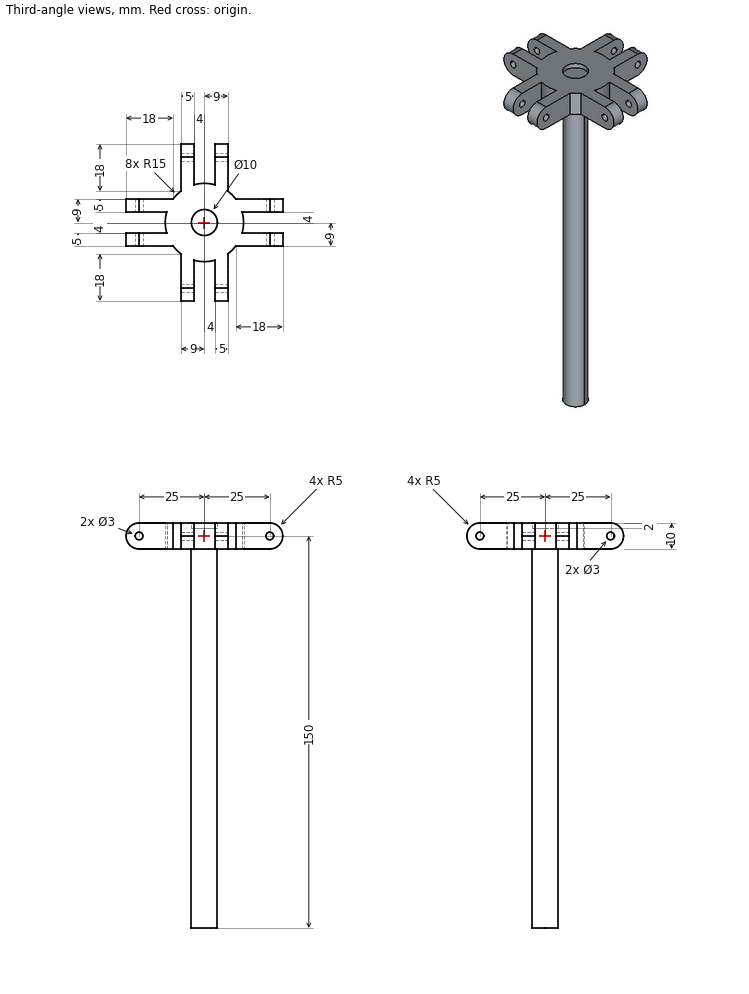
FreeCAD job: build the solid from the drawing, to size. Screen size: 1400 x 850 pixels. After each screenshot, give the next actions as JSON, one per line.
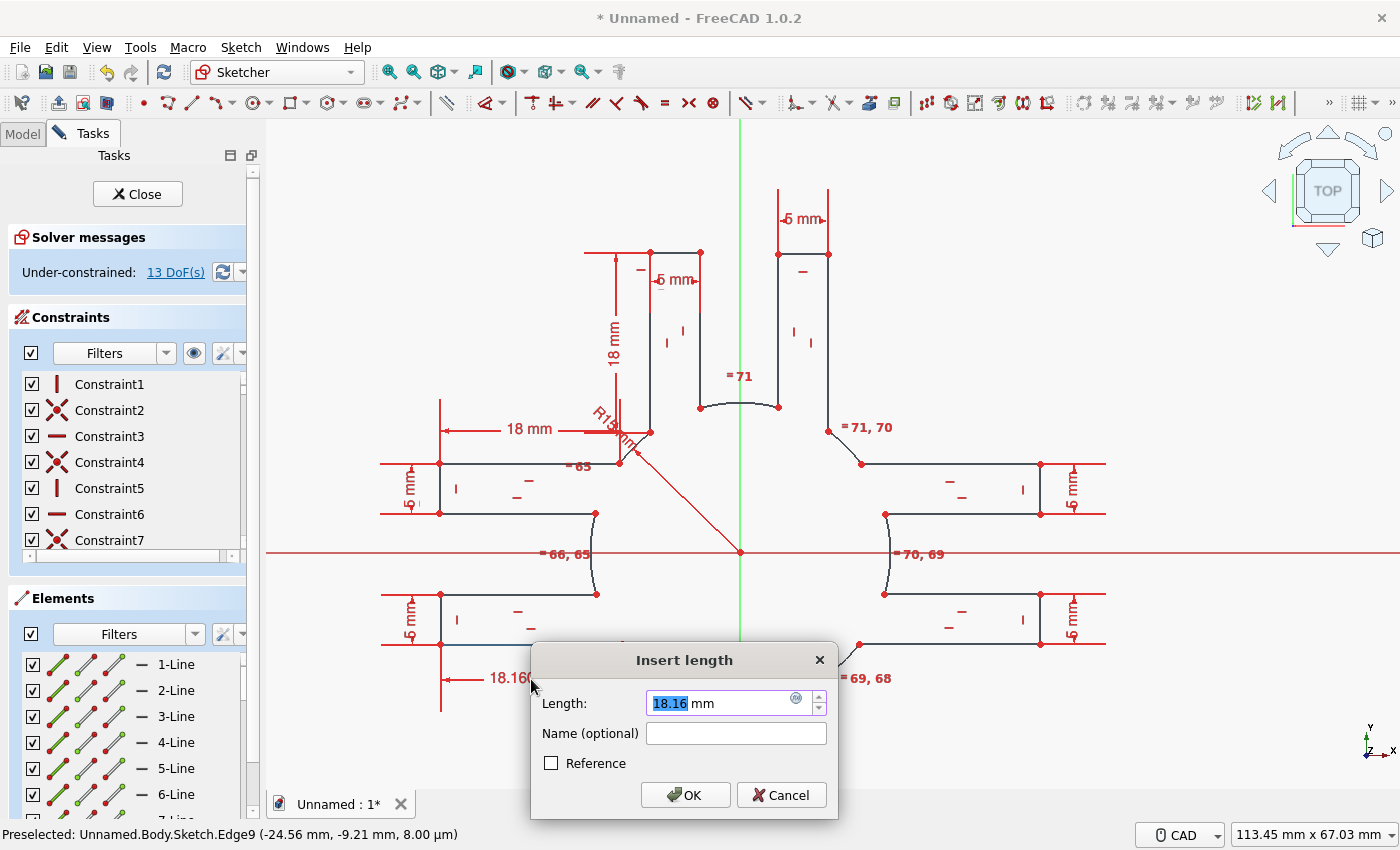
{"action": "type", "text": "18"}
{"action": "key", "text": "Return"}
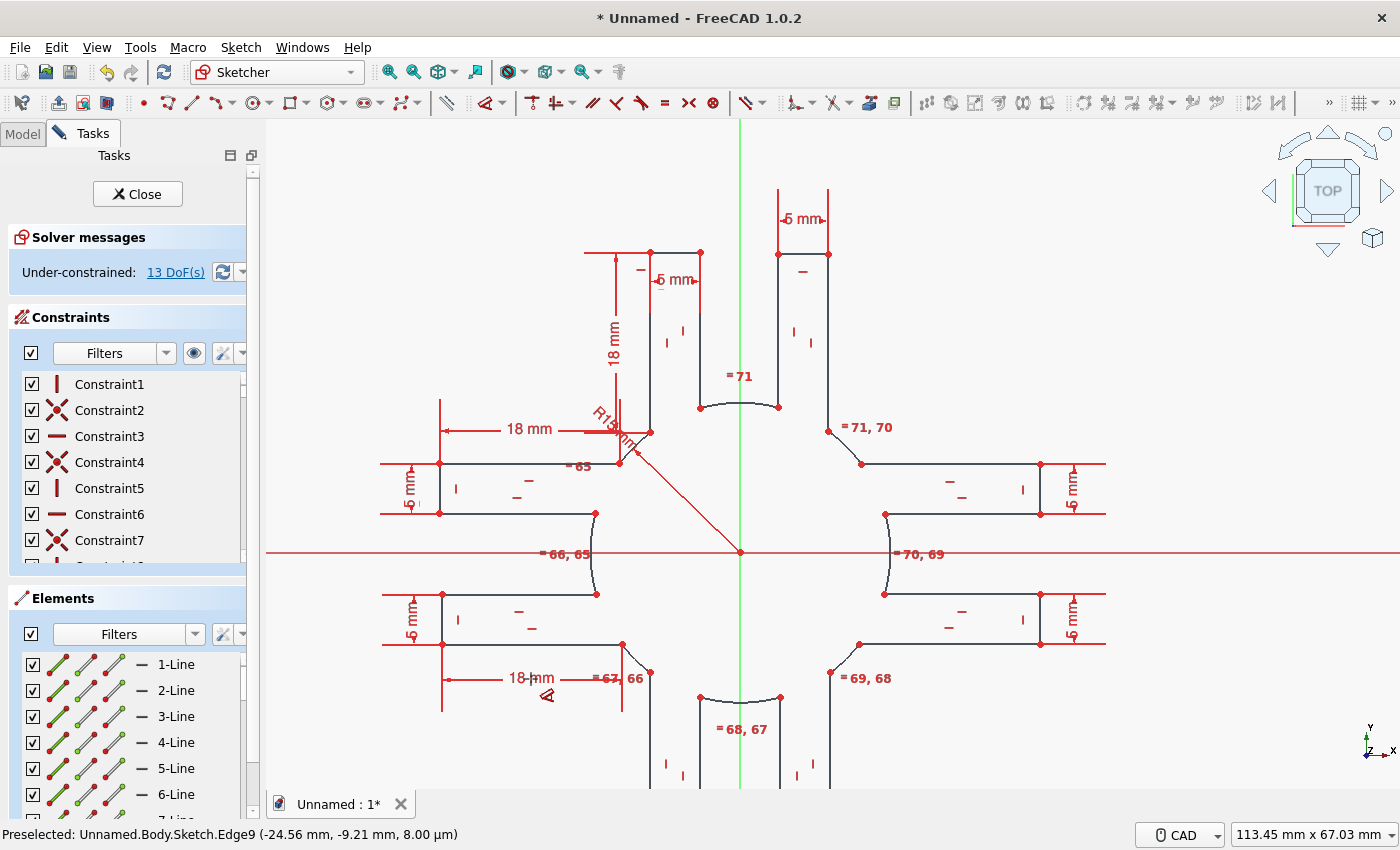
{"action": "left_click", "coordinate": [650, 727]}
{"action": "left_click", "coordinate": [616, 717]}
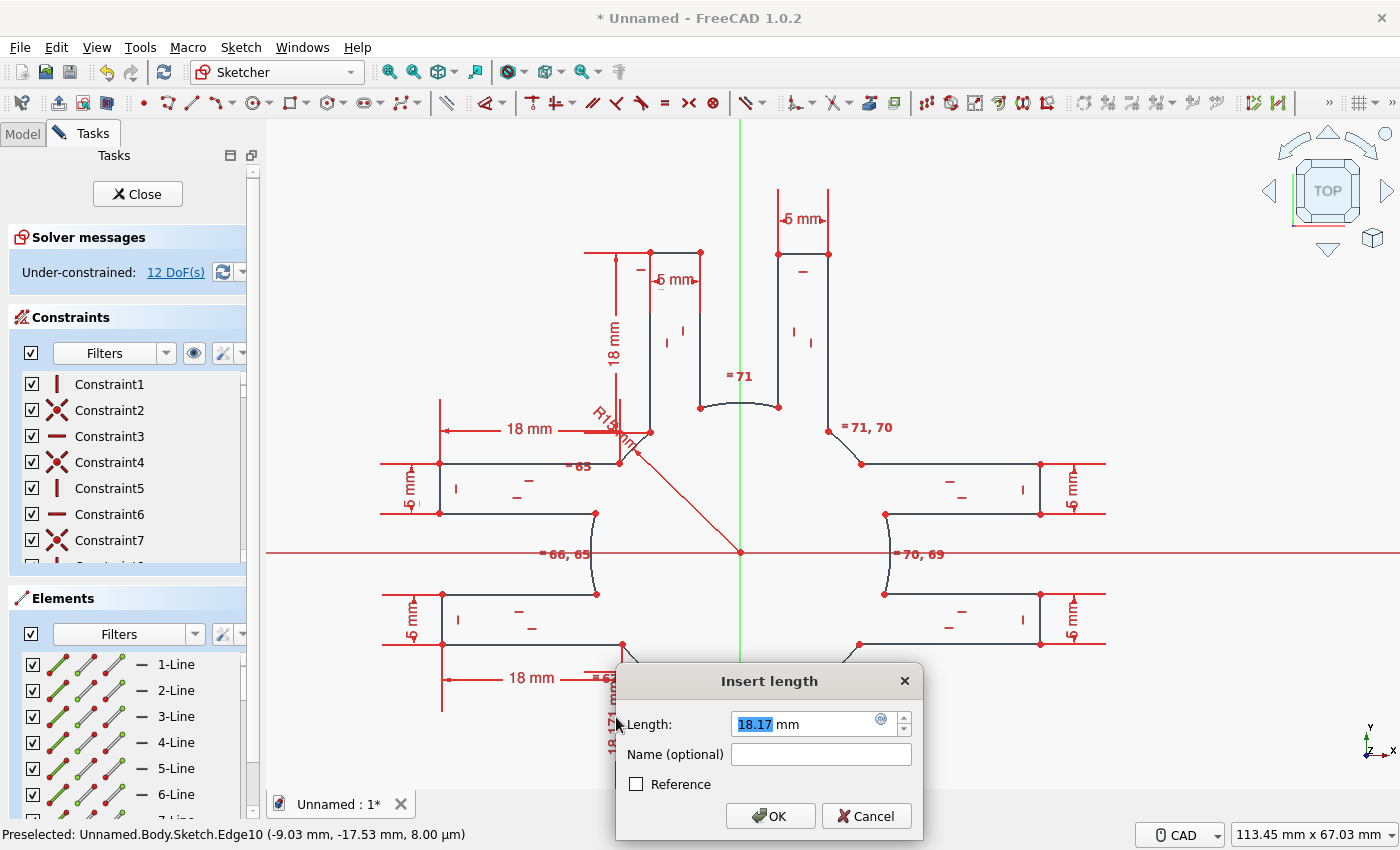
{"action": "type", "text": "18"}
{"action": "key", "text": "Return"}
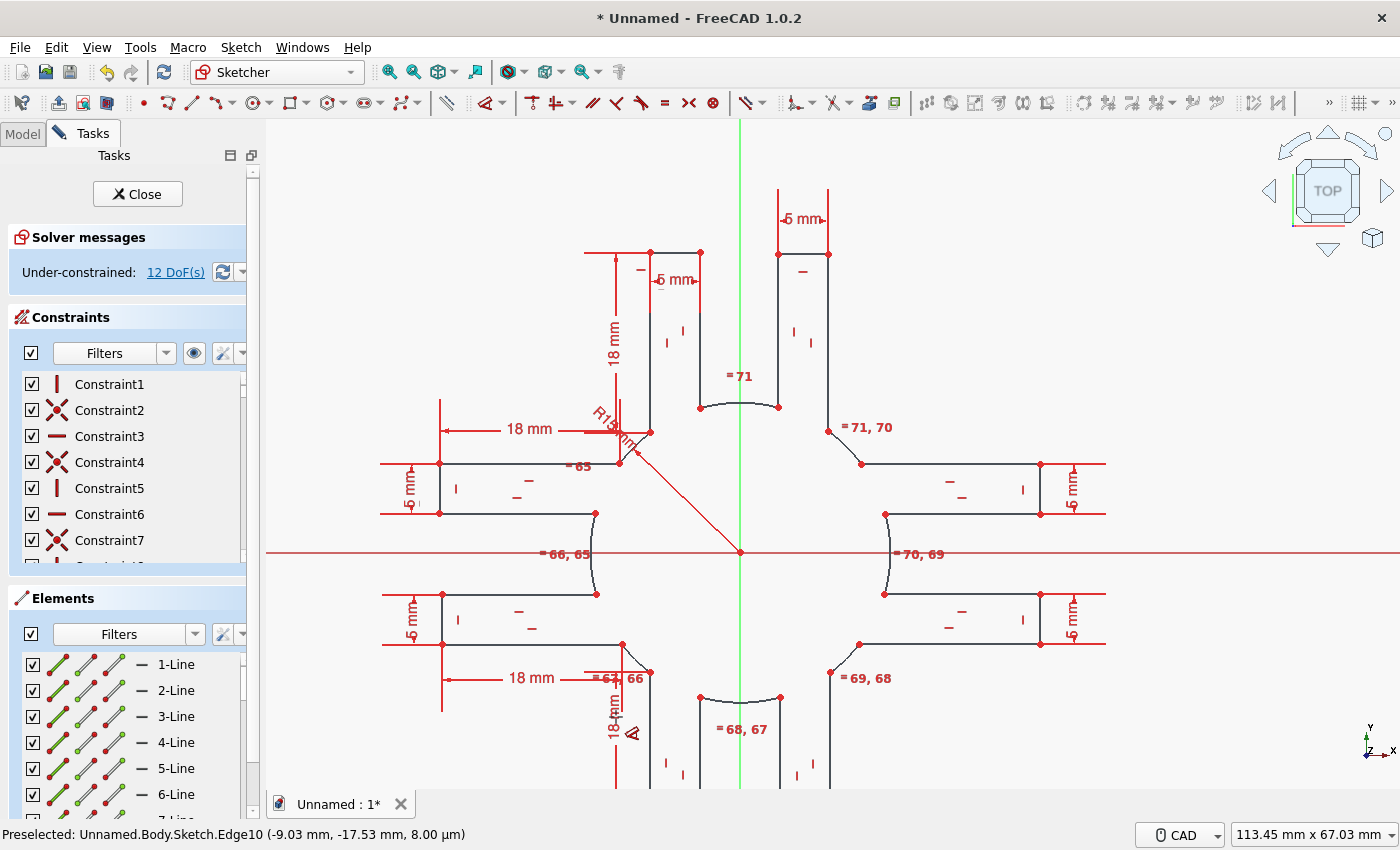
{"action": "left_click", "coordinate": [830, 727]}
{"action": "left_click", "coordinate": [864, 717]}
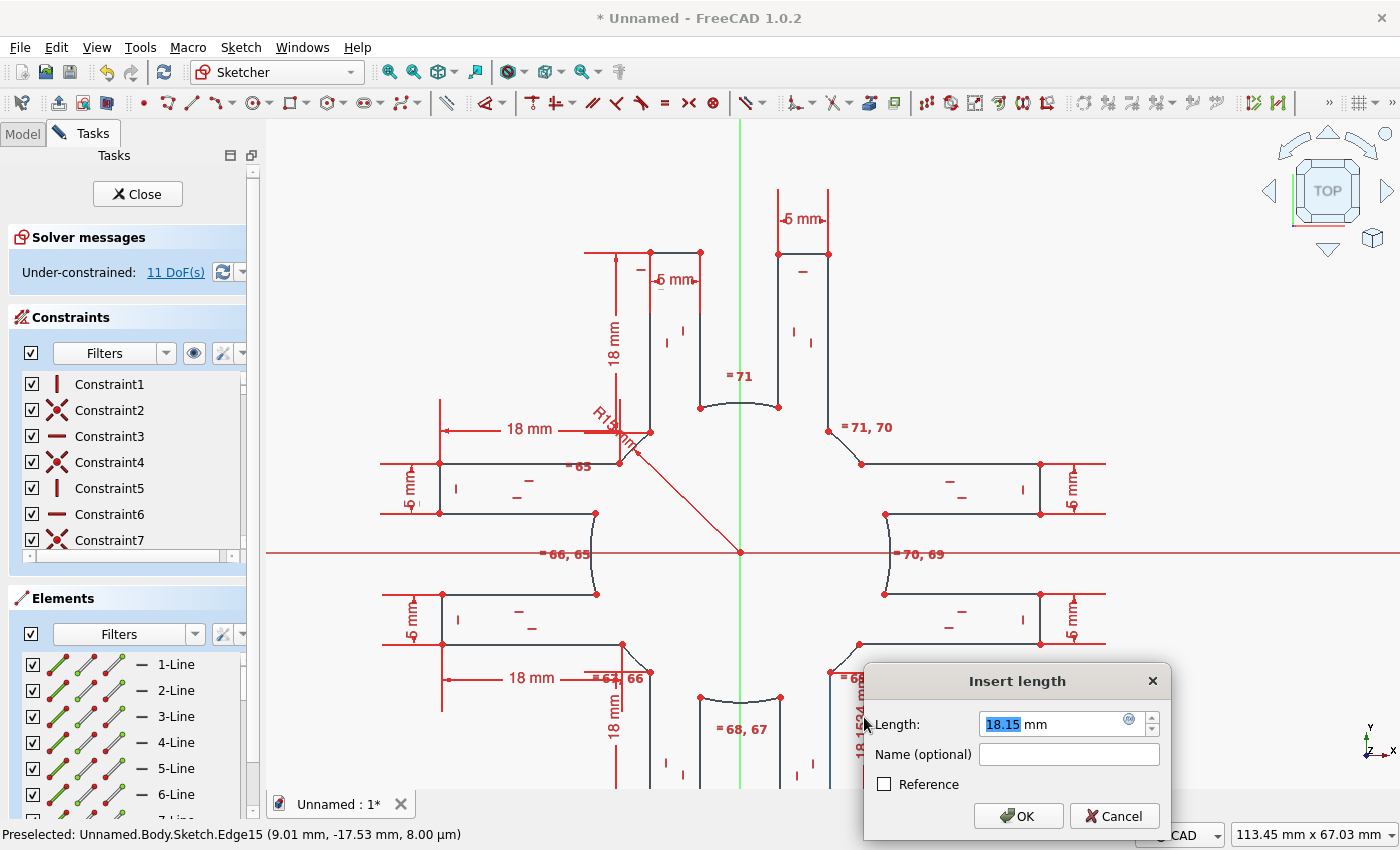
{"action": "type", "text": "18"}
{"action": "key", "text": "Return"}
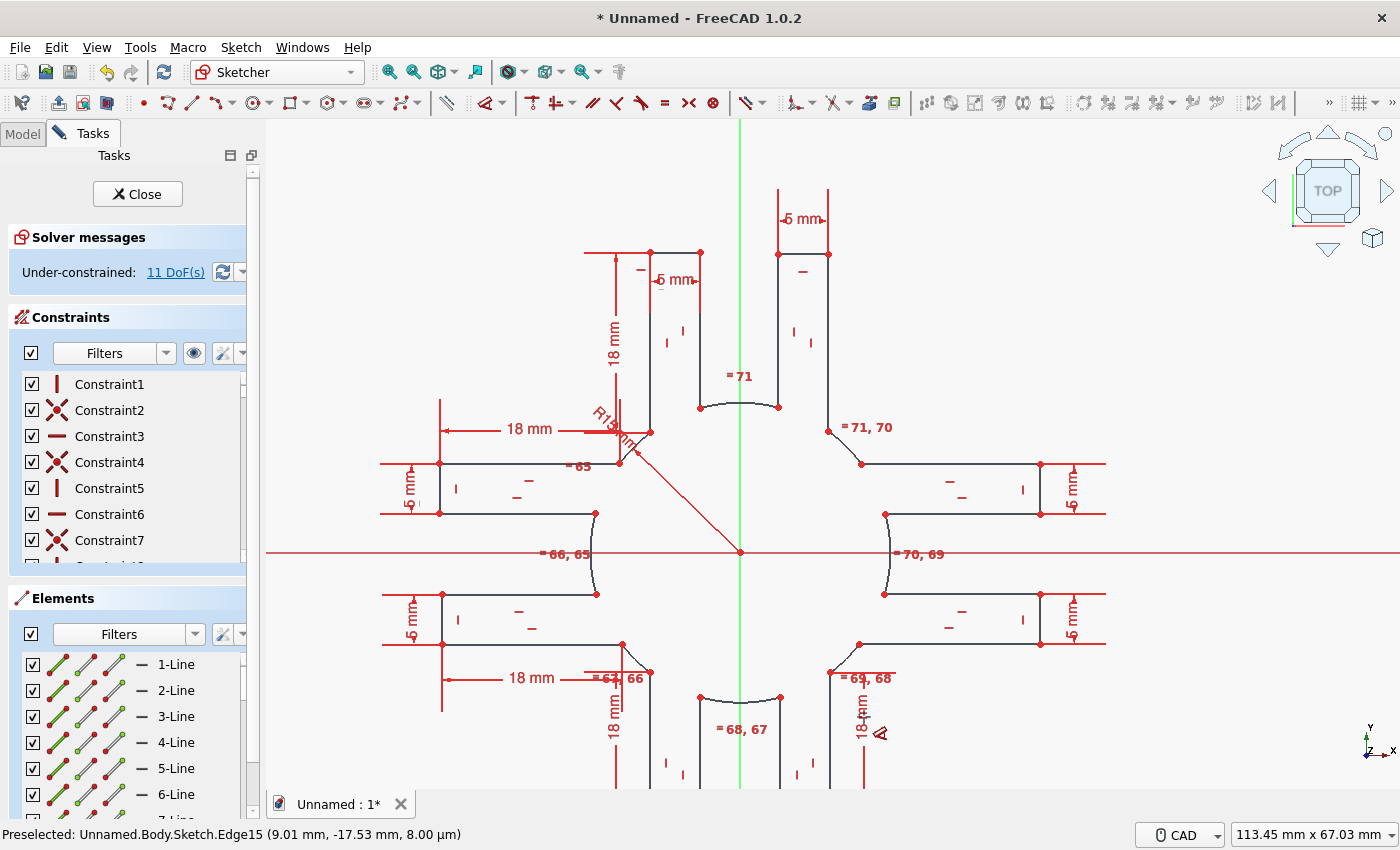
{"action": "left_click", "coordinate": [914, 644]}
{"action": "left_click", "coordinate": [950, 678]}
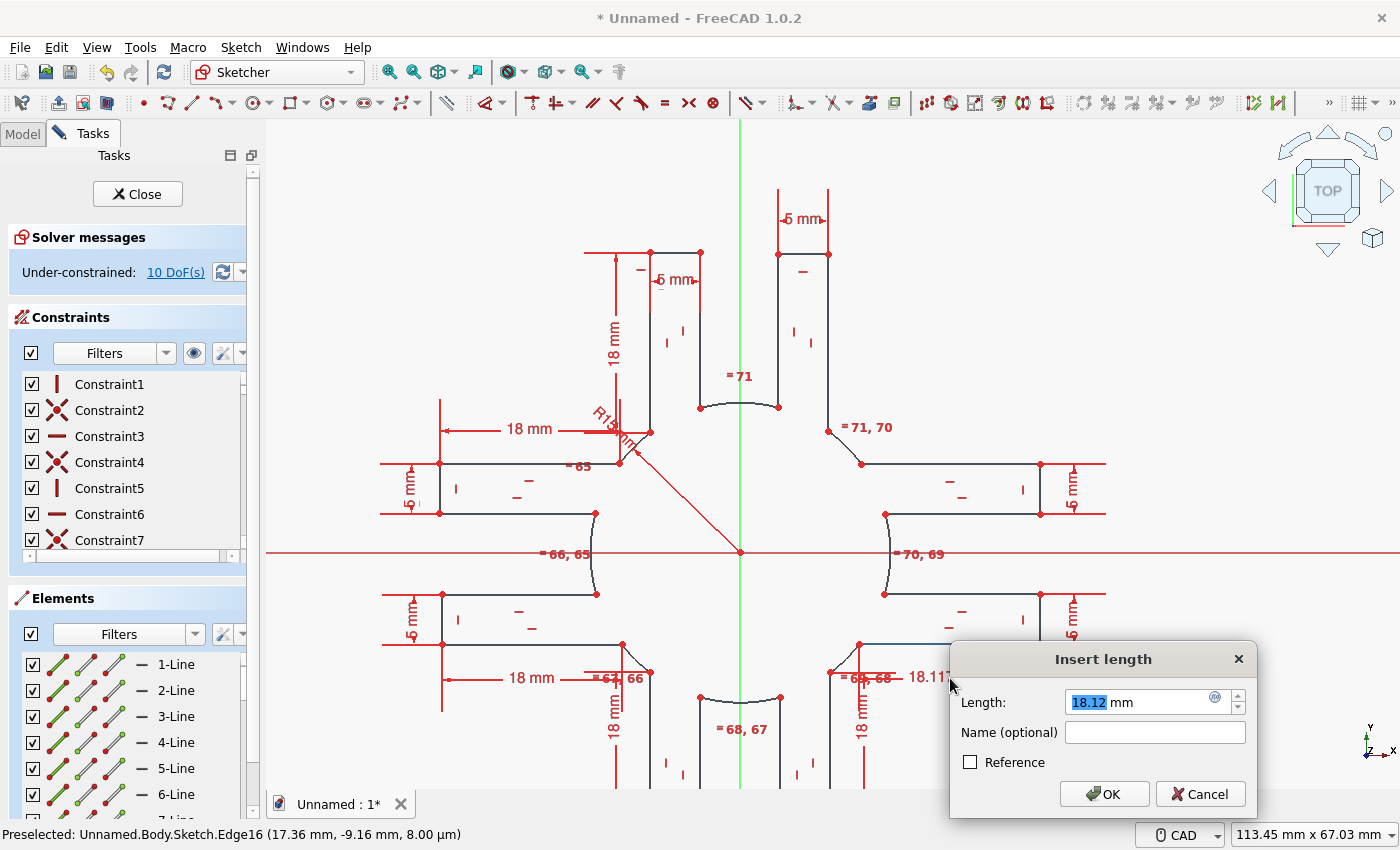
{"action": "type", "text": "18"}
{"action": "key", "text": "Return"}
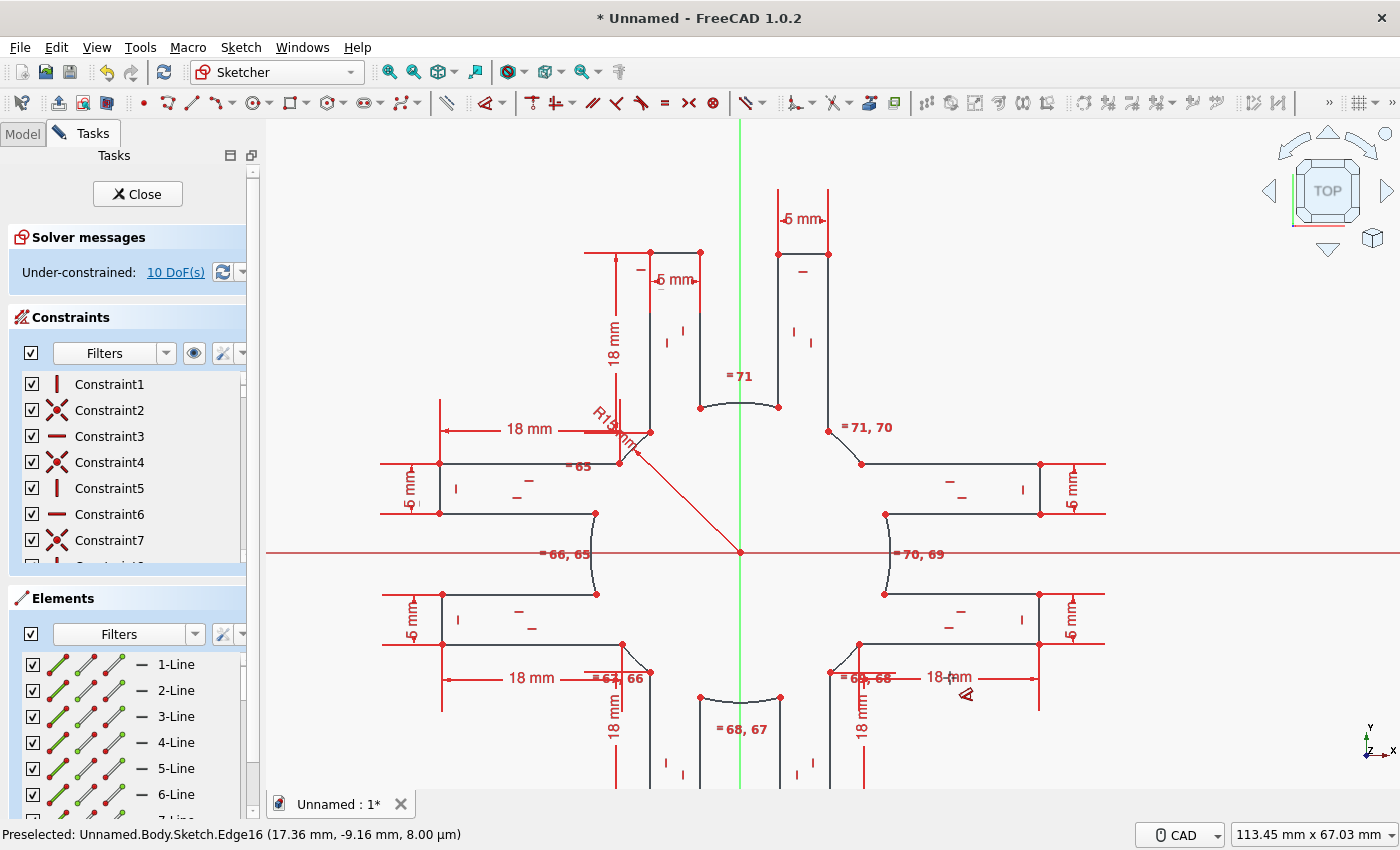
{"action": "left_click", "coordinate": [987, 464]}
{"action": "left_click", "coordinate": [951, 430]}